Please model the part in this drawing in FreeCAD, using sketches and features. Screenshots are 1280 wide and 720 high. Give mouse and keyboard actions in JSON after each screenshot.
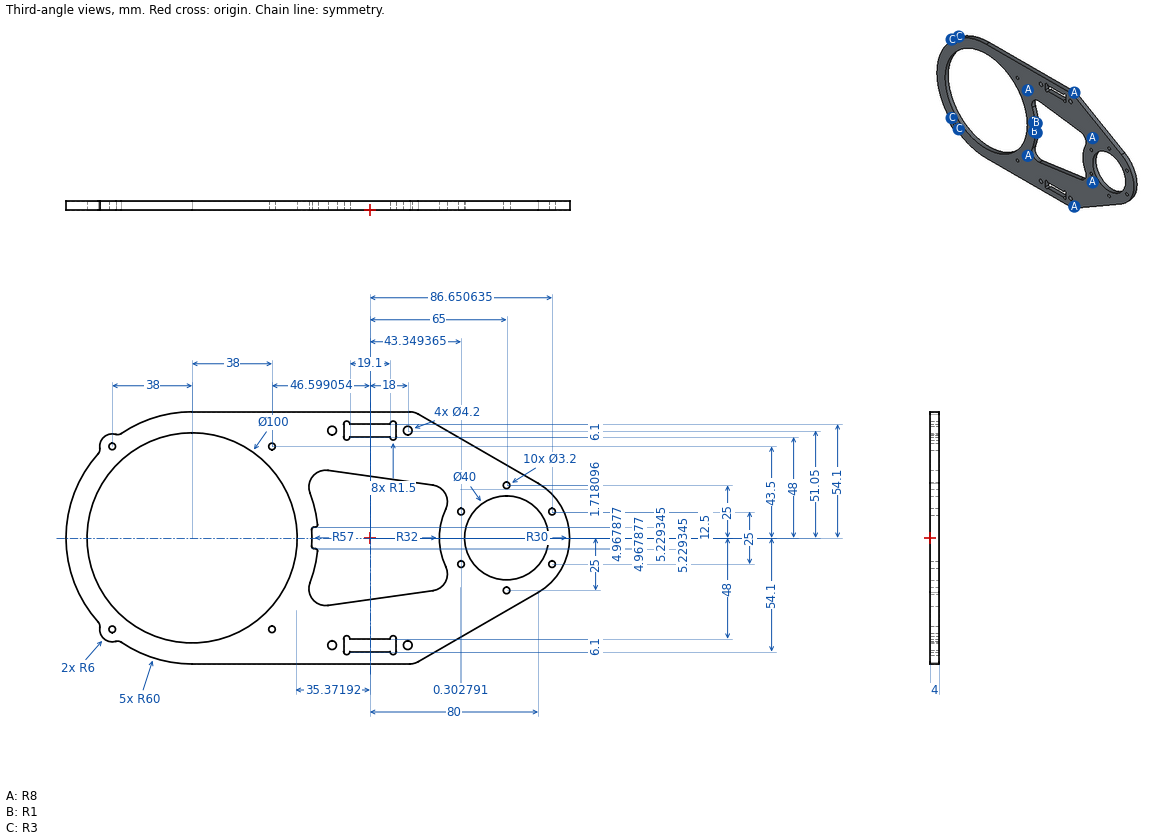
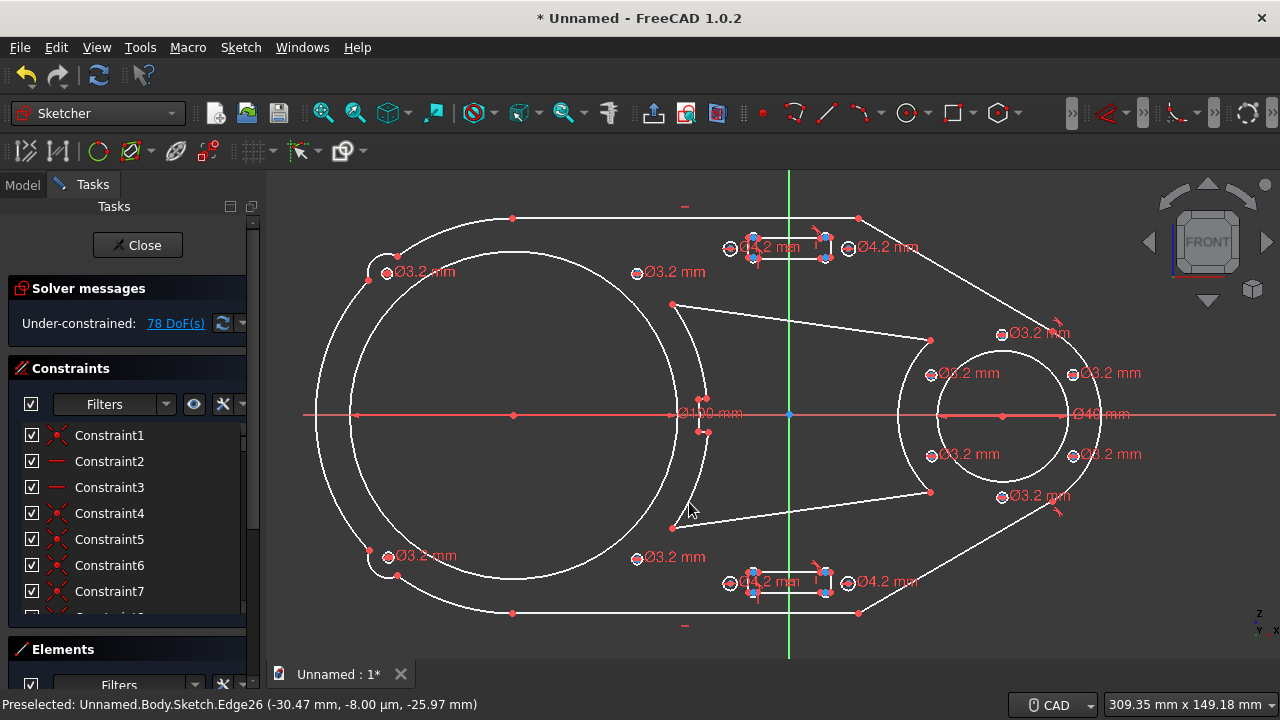
{"action": "left_click", "coordinate": [429, 595]}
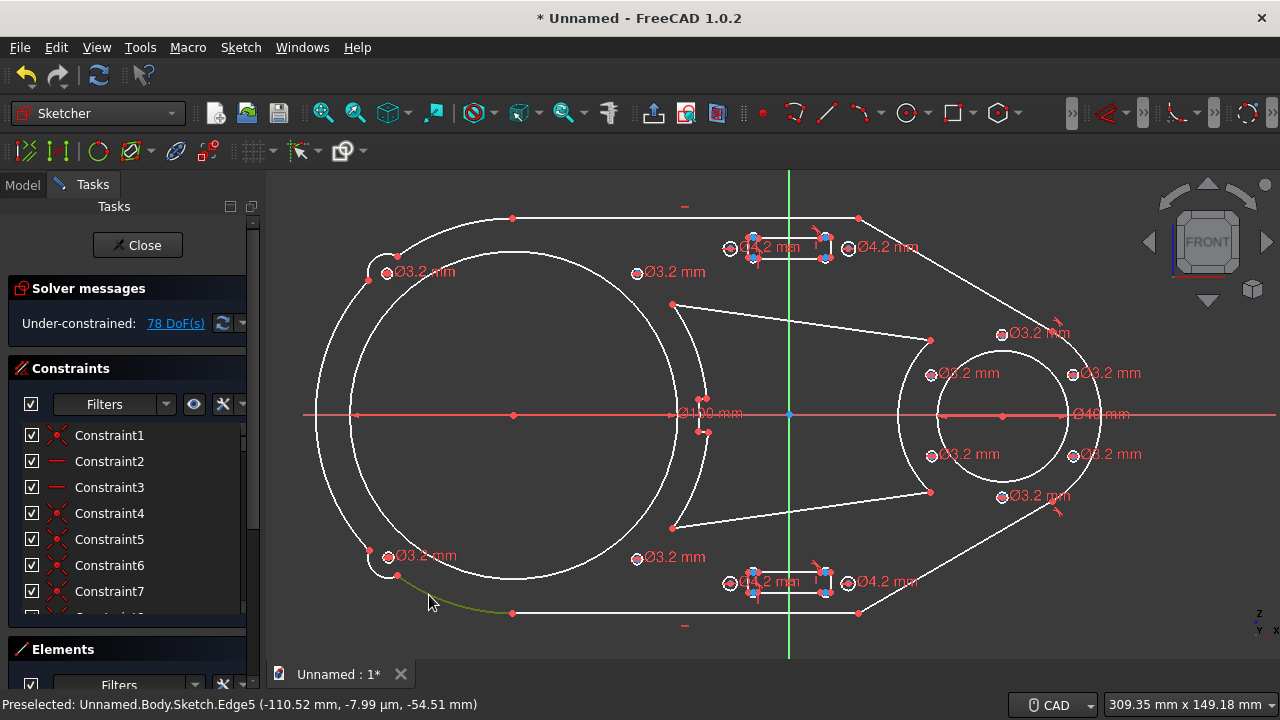
{"action": "left_click", "coordinate": [325, 357]}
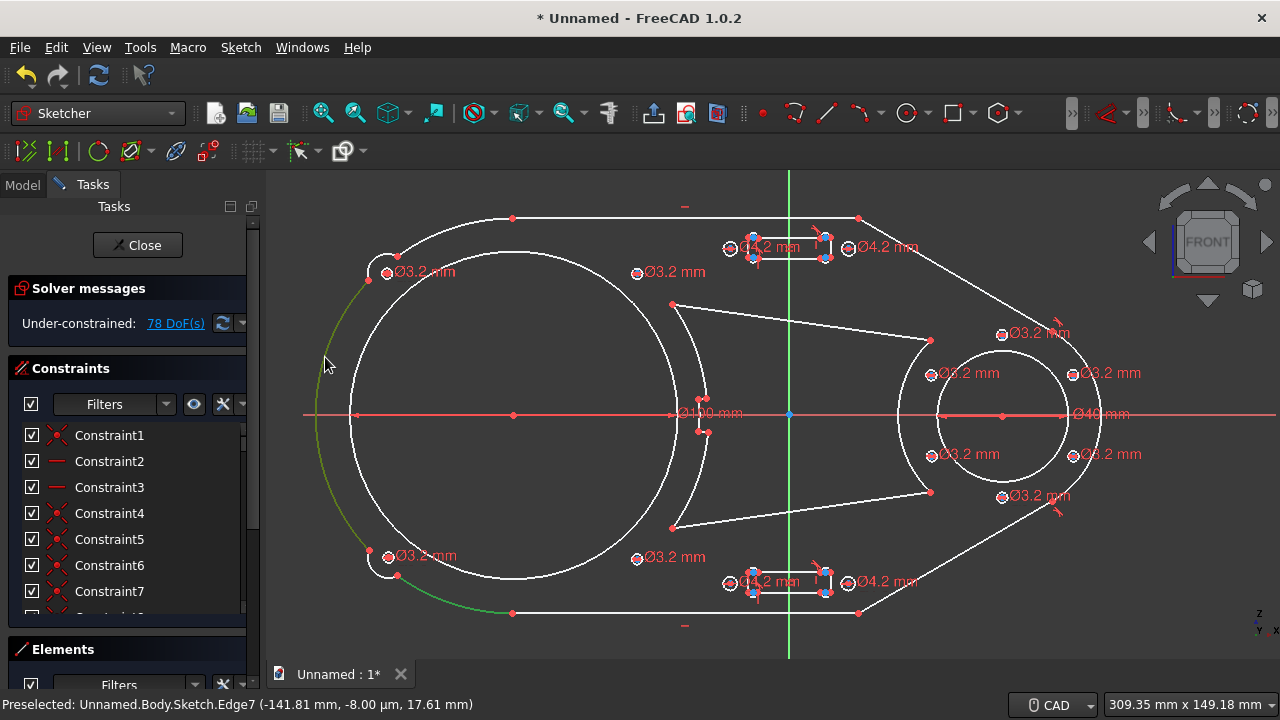
{"action": "left_click", "coordinate": [476, 222]}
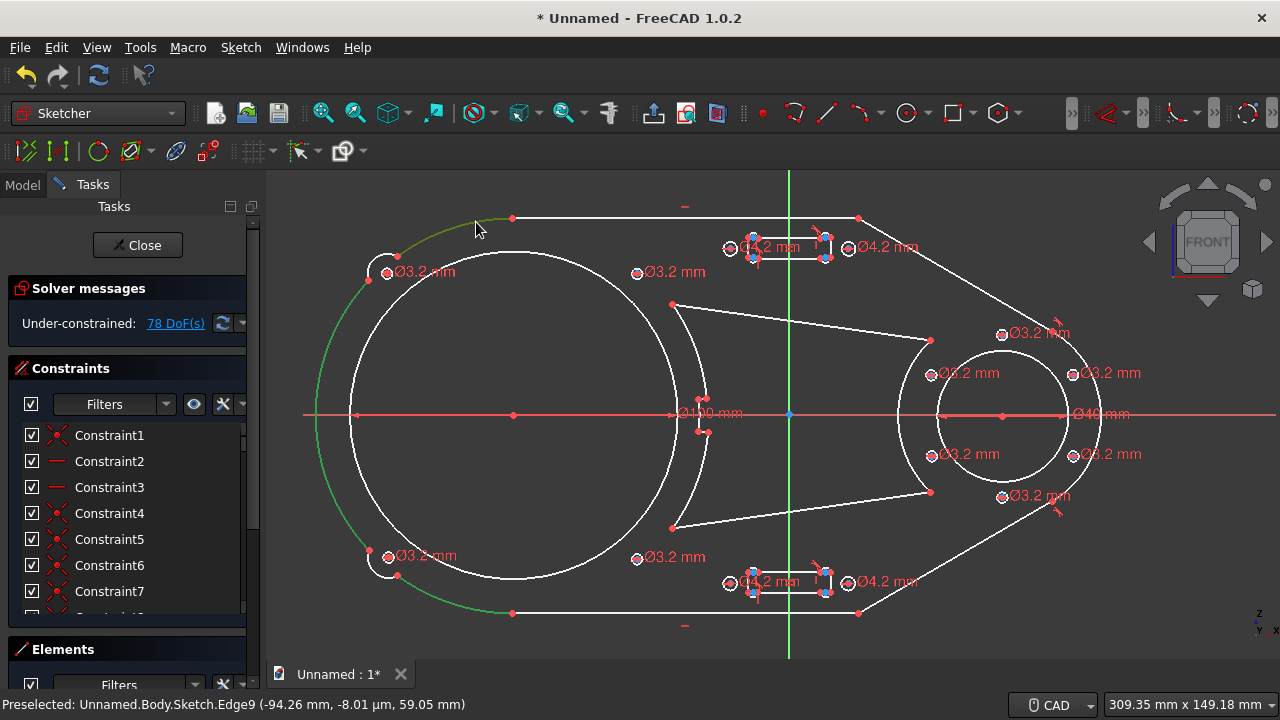
{"action": "left_click", "coordinate": [702, 369]}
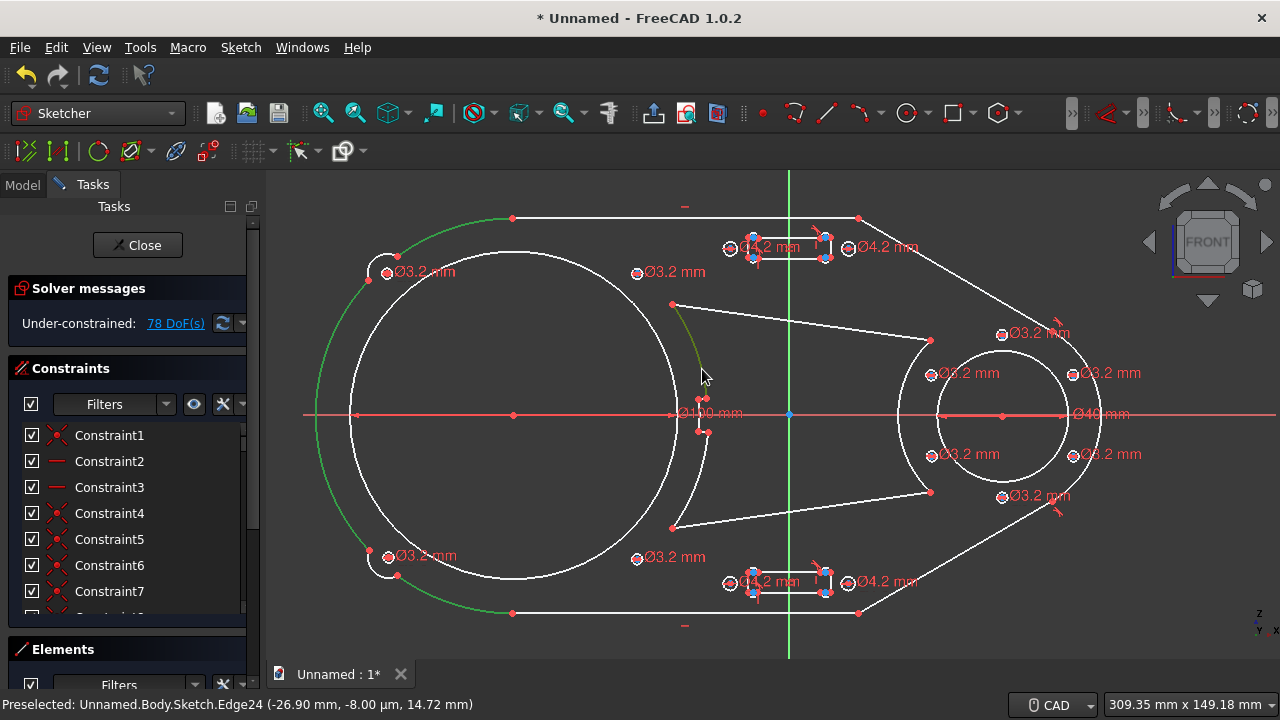
{"action": "left_click", "coordinate": [689, 502]}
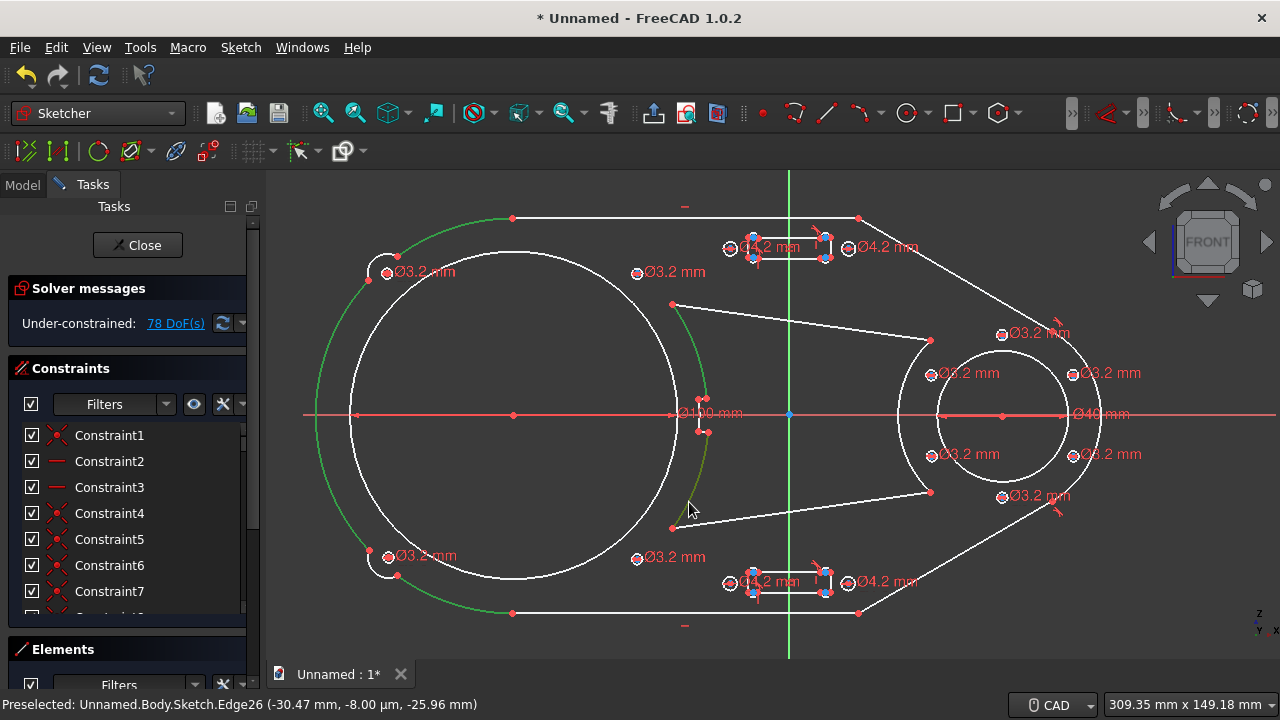
{"action": "key", "text": "e"}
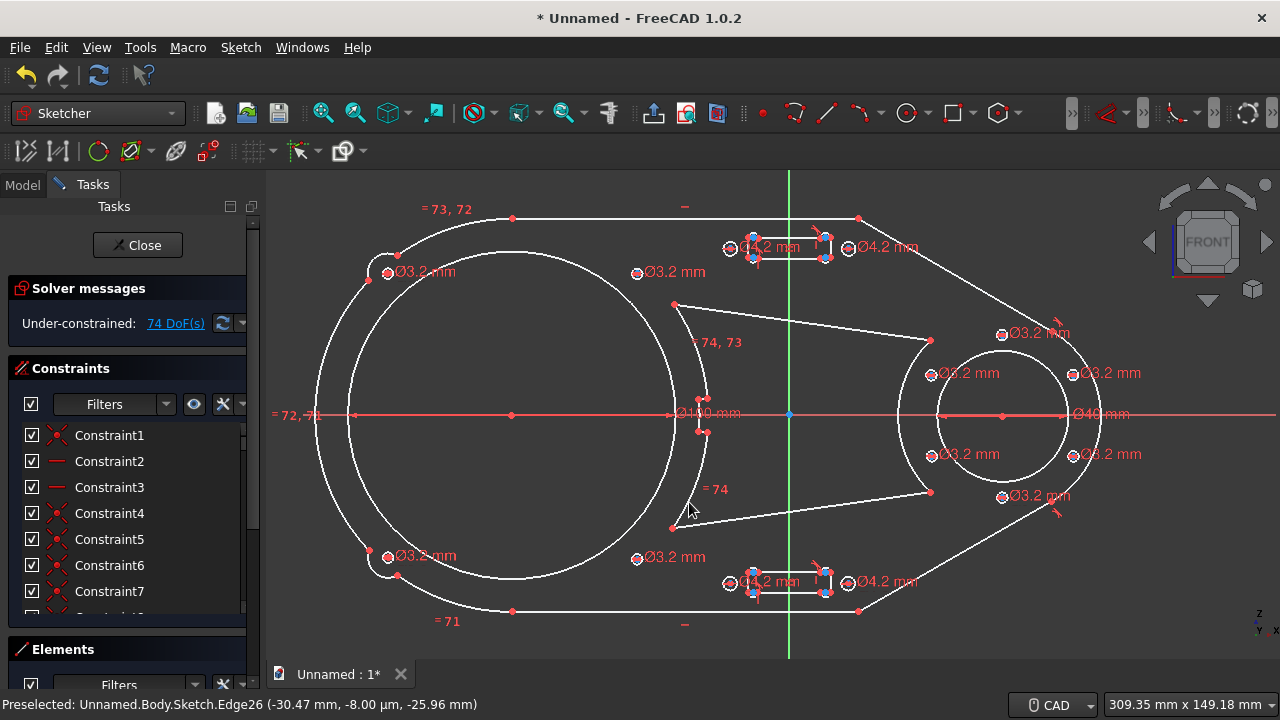
{"action": "left_click", "coordinate": [370, 565]}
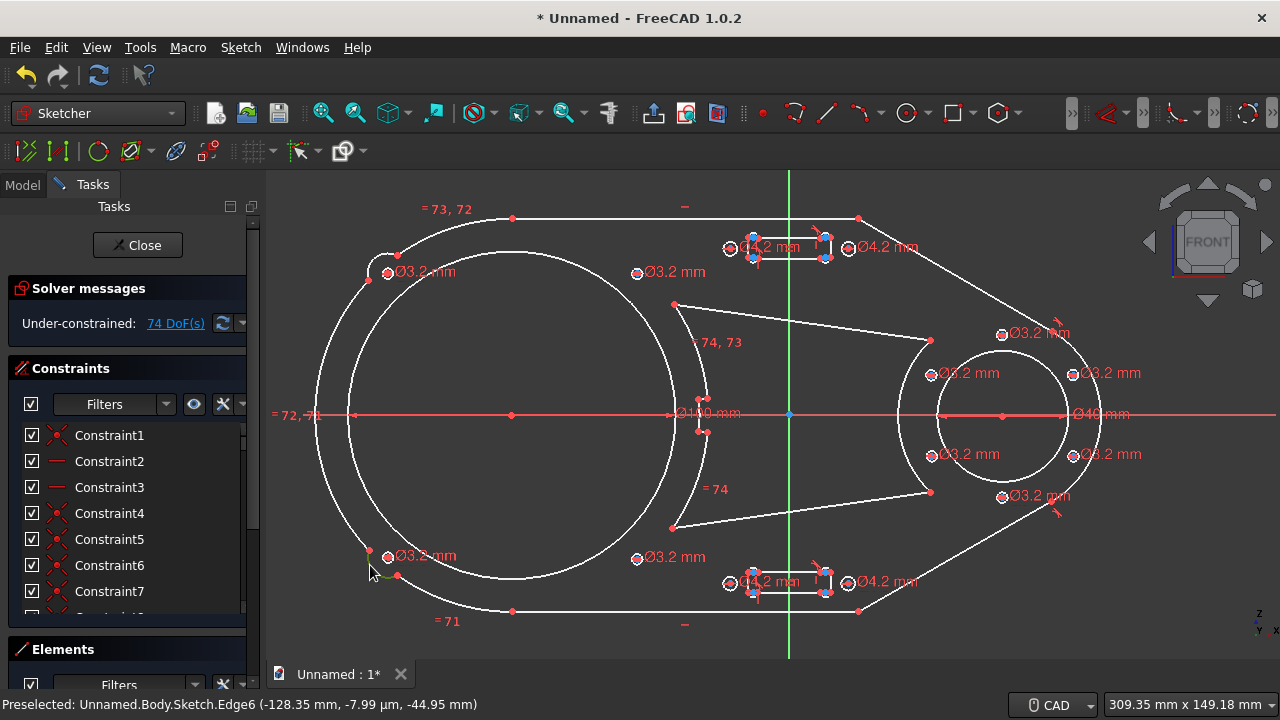
{"action": "left_click", "coordinate": [383, 254]}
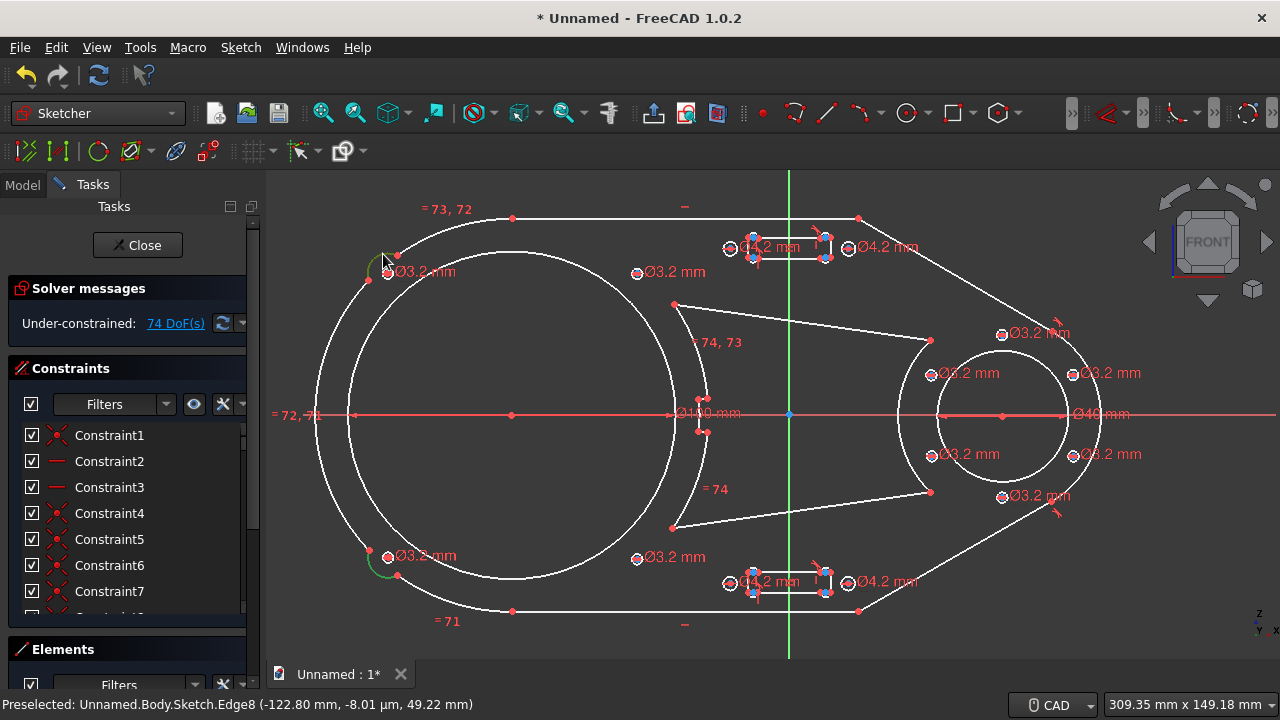
{"action": "key", "text": "e"}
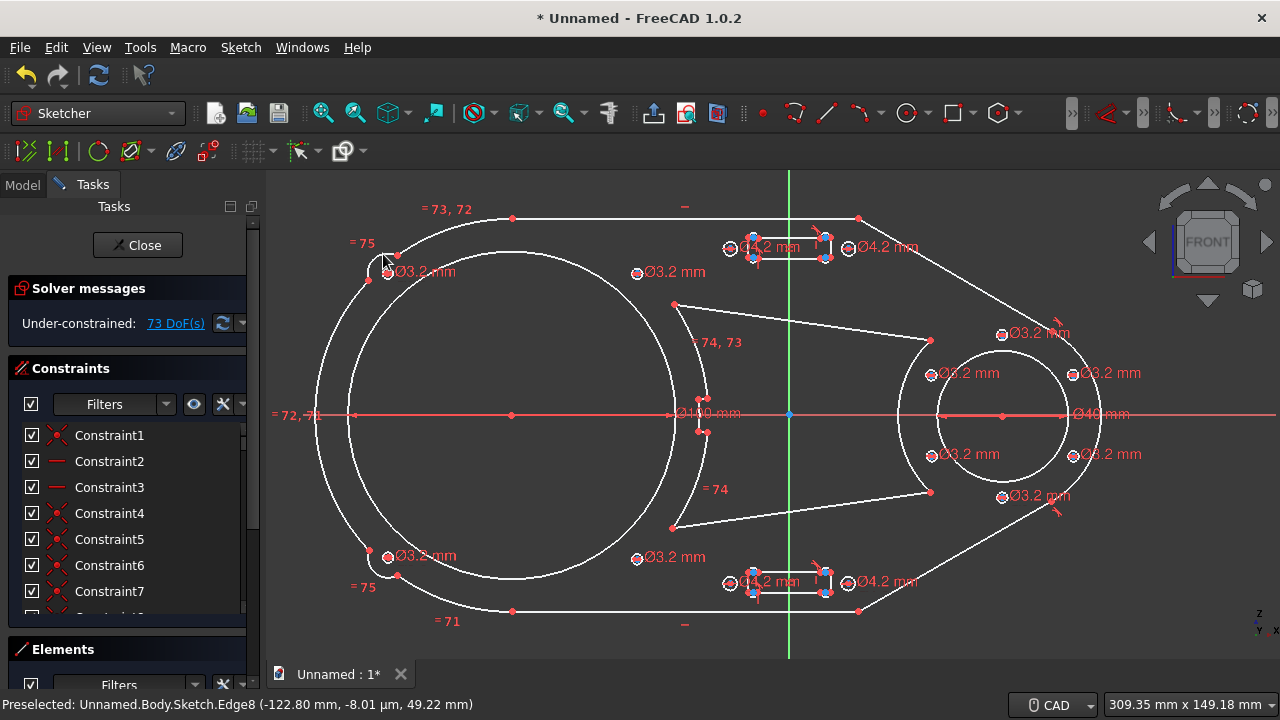
{"action": "scroll", "coordinate": [826, 263], "scroll_direction": "up", "scroll_amount": 6}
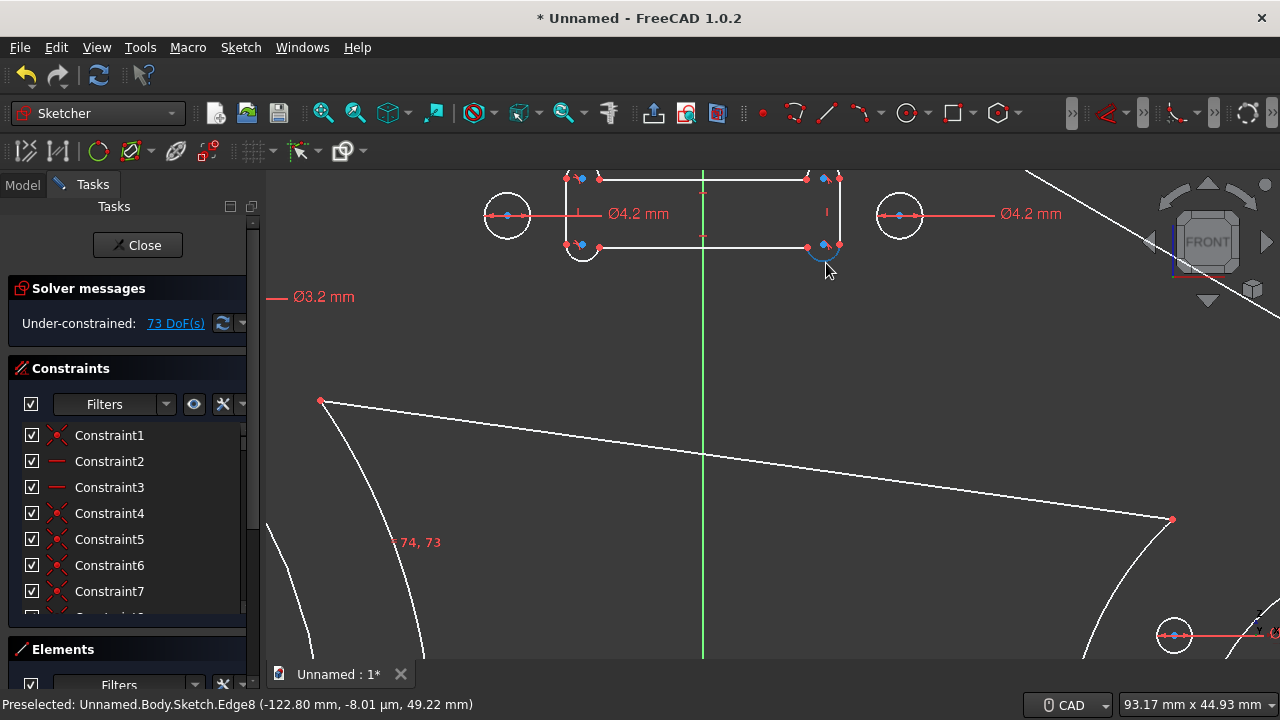
{"action": "left_click", "coordinate": [825, 261]}